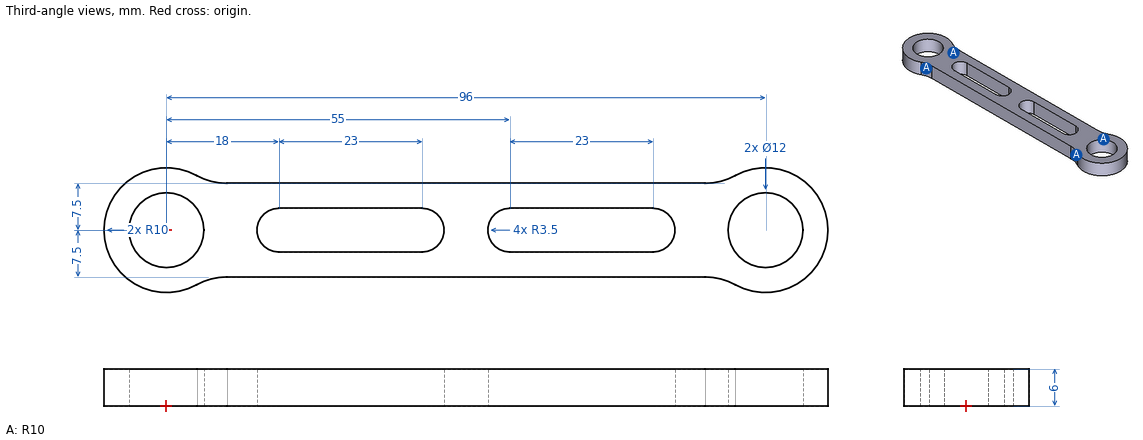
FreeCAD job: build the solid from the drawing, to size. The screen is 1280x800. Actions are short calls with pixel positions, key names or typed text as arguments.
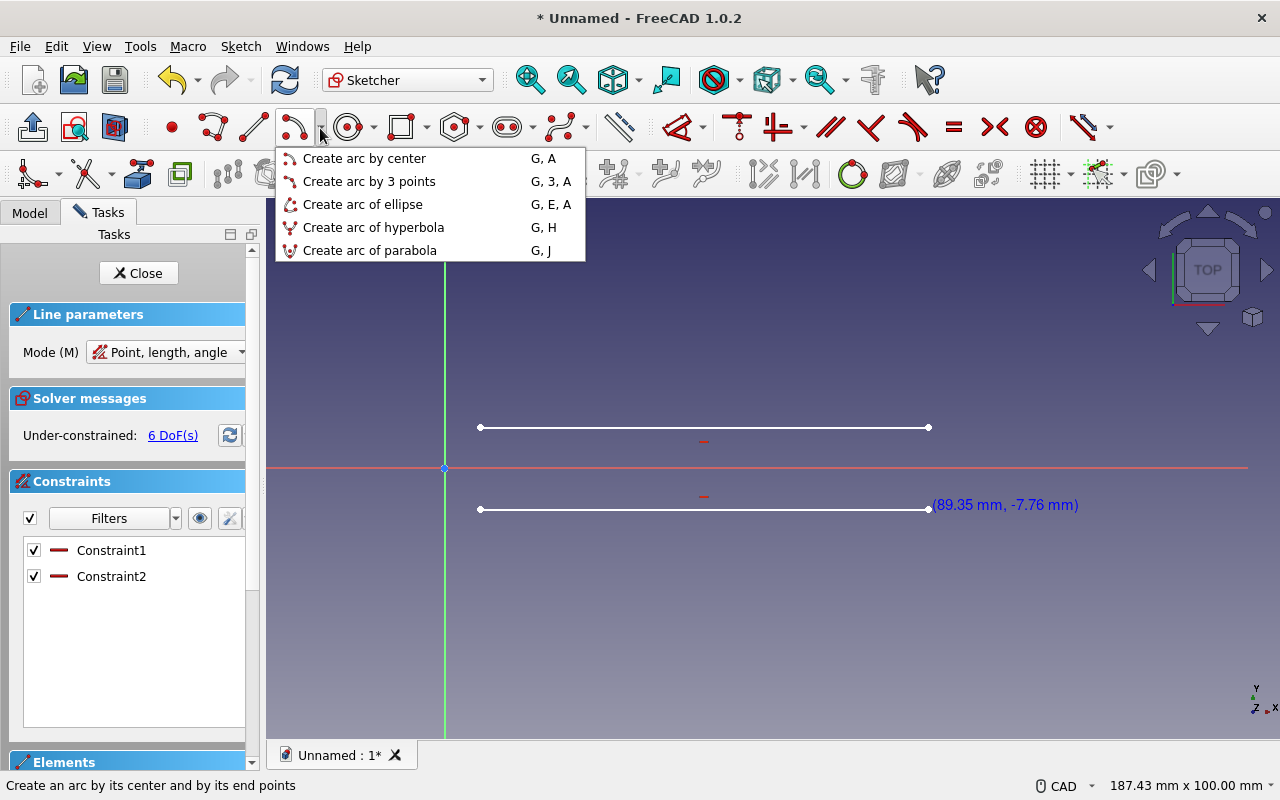
click(430, 182)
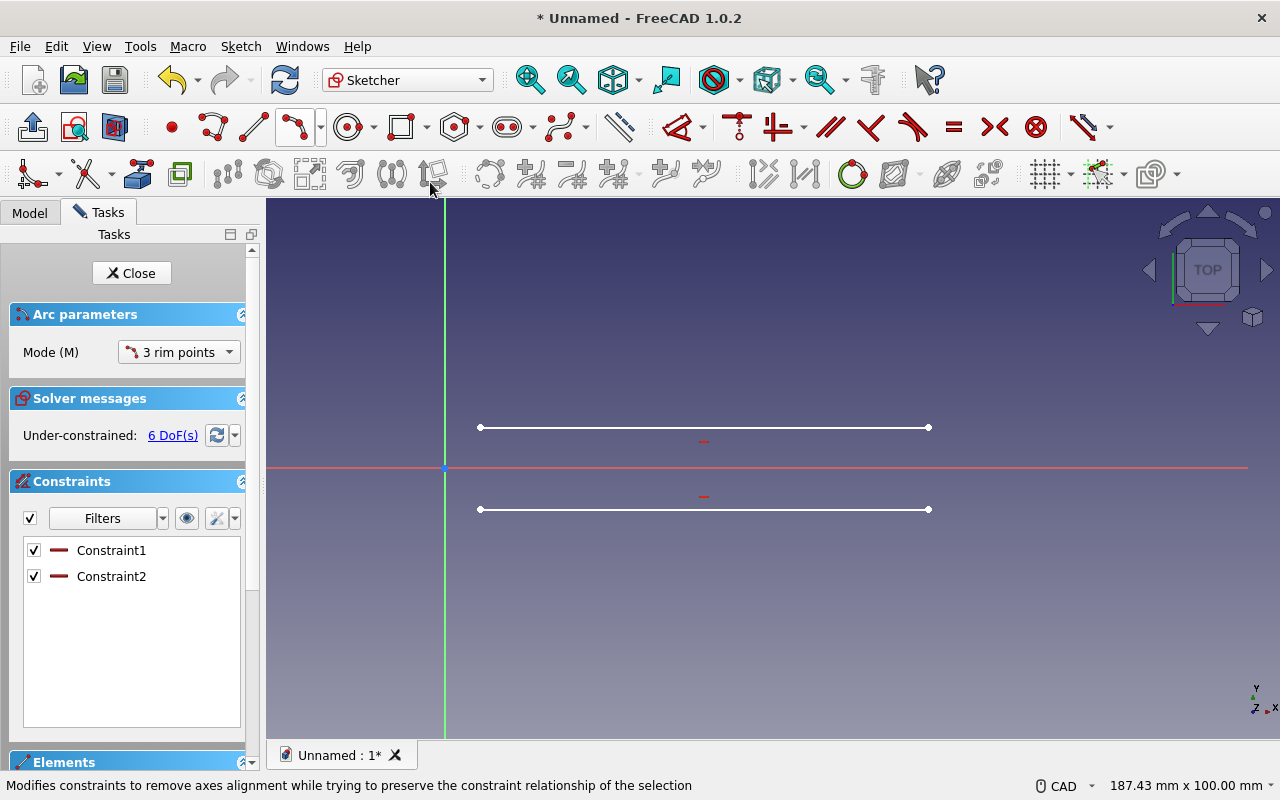
click(480, 428)
click(480, 510)
click(396, 444)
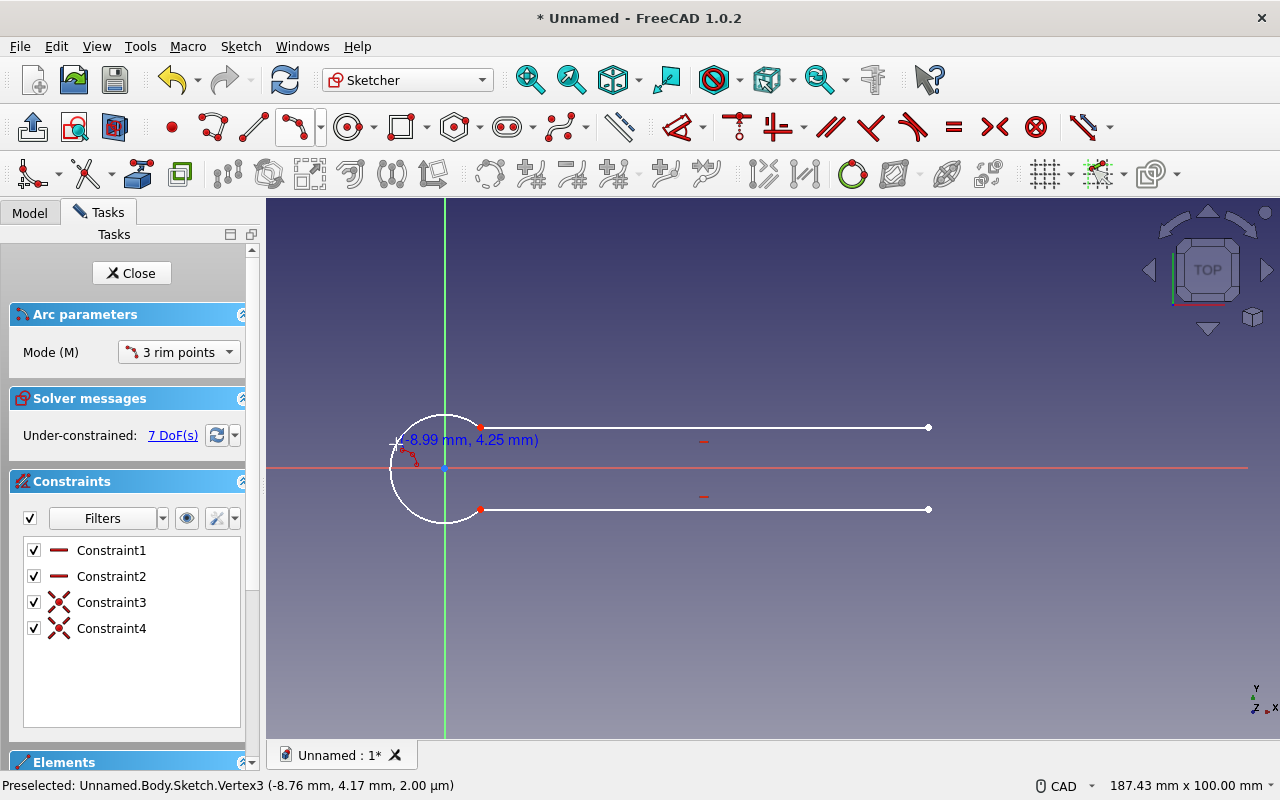
click(928, 510)
click(928, 428)
click(1012, 492)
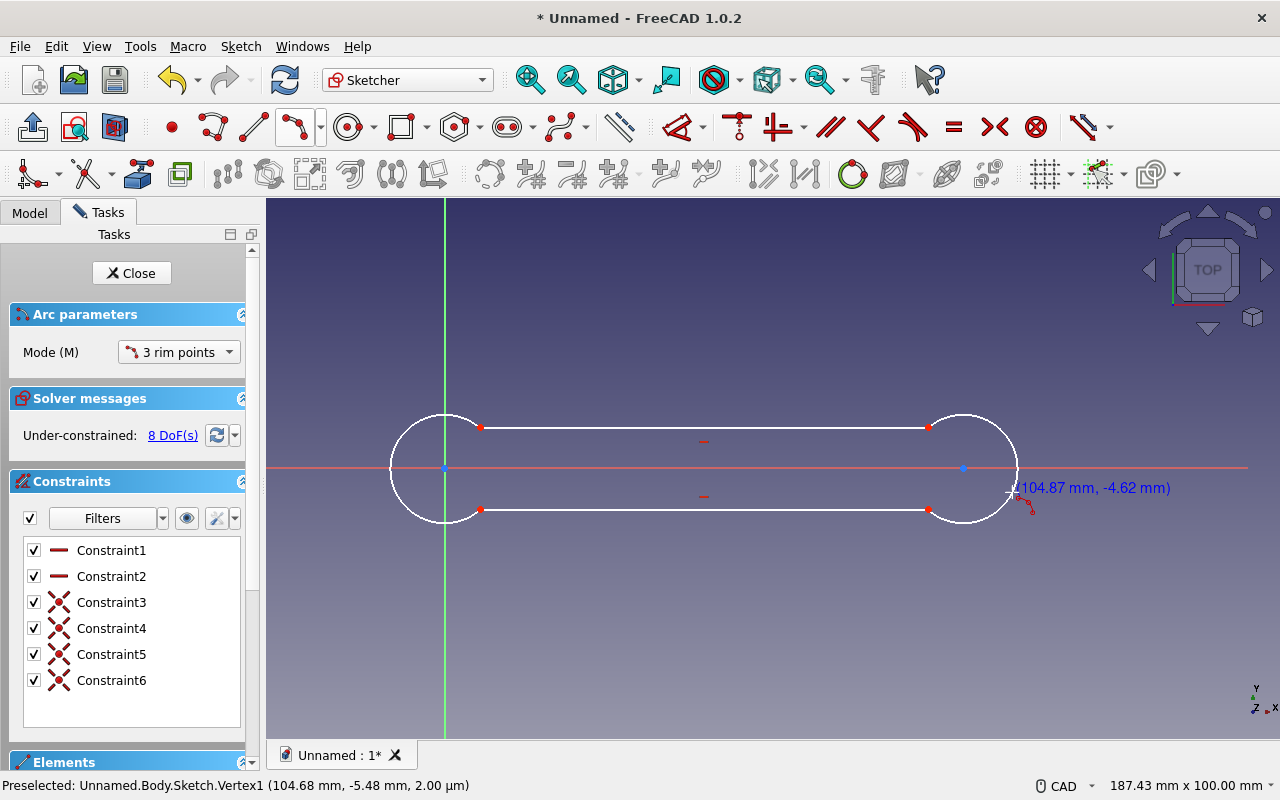
key(g)
key(s)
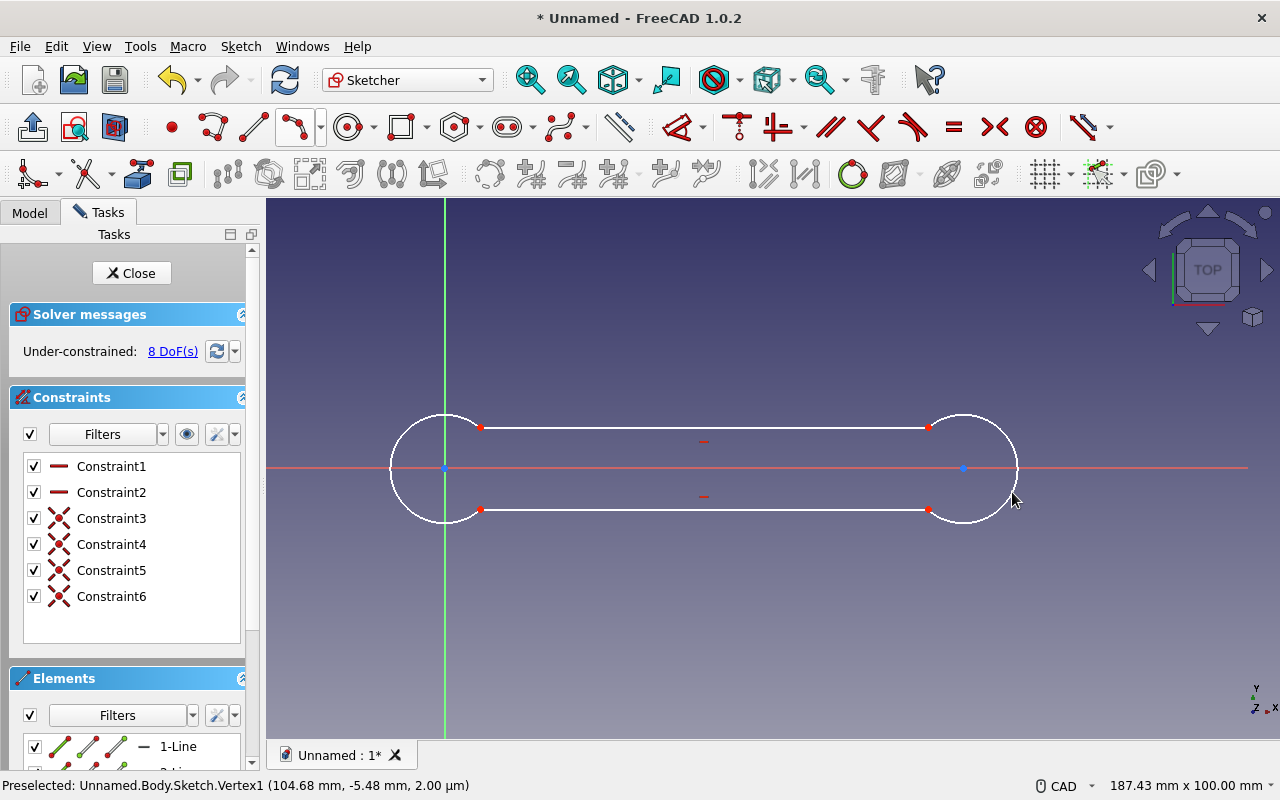
click(742, 468)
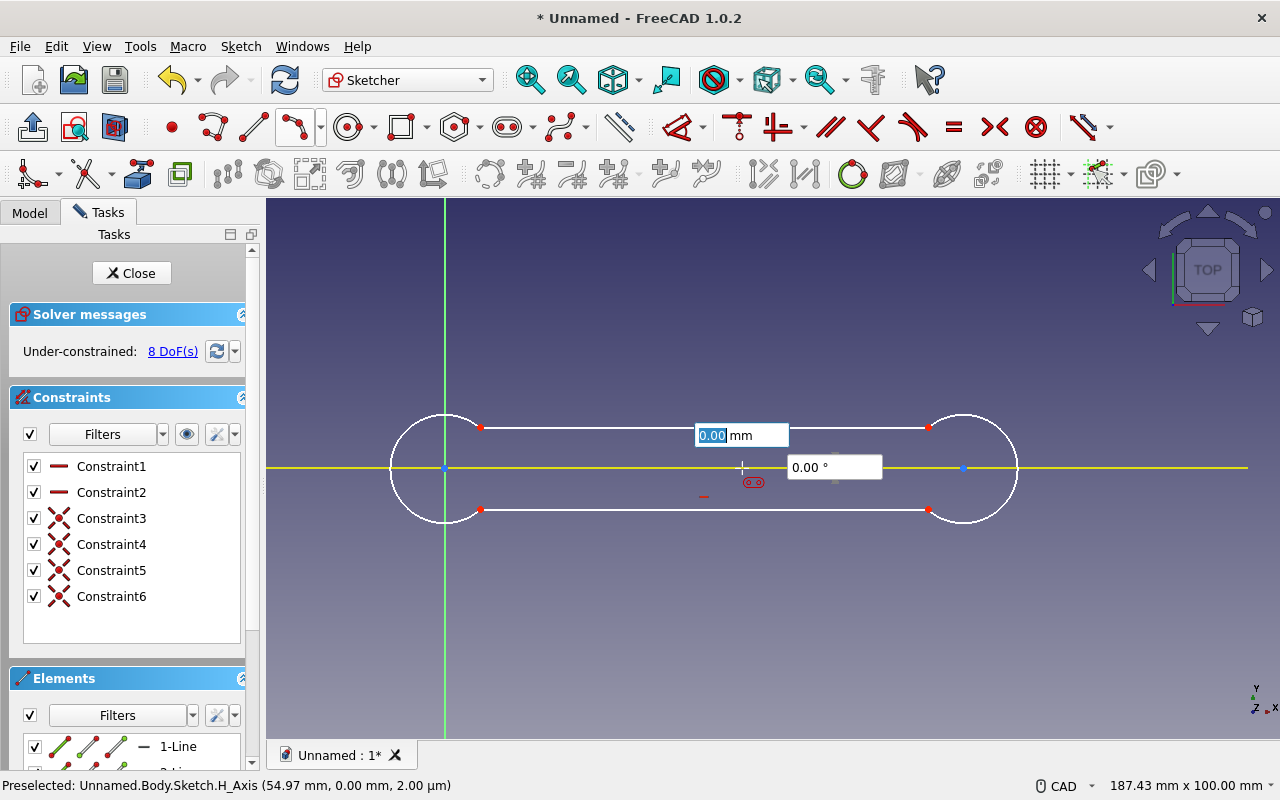
click(867, 459)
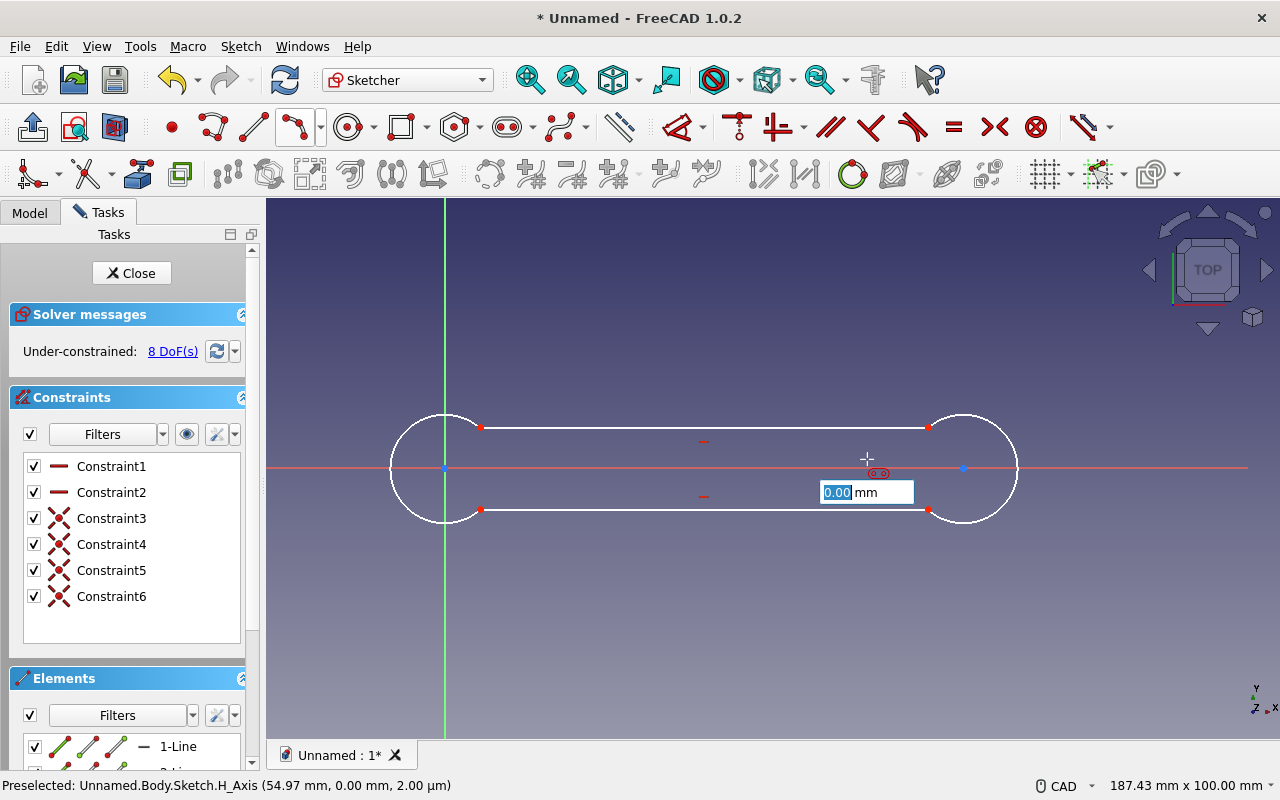
click(804, 487)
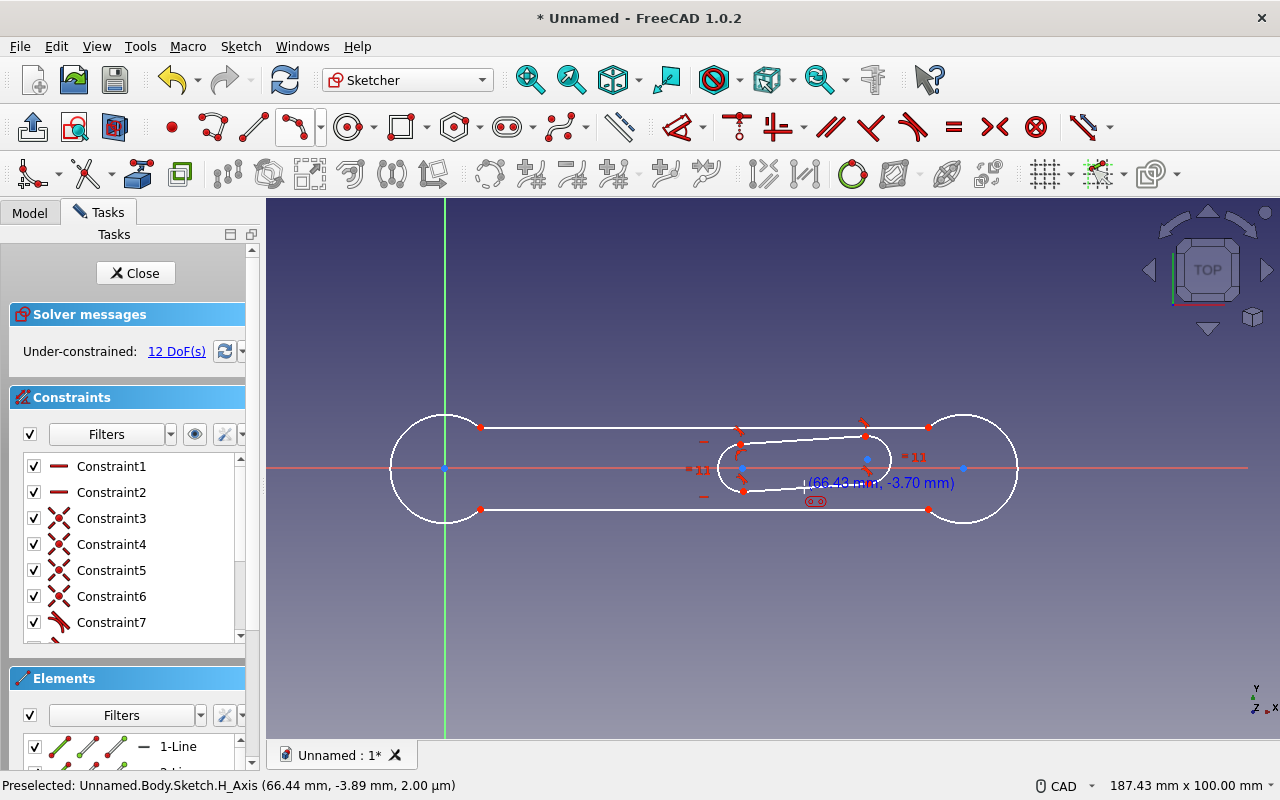
click(542, 468)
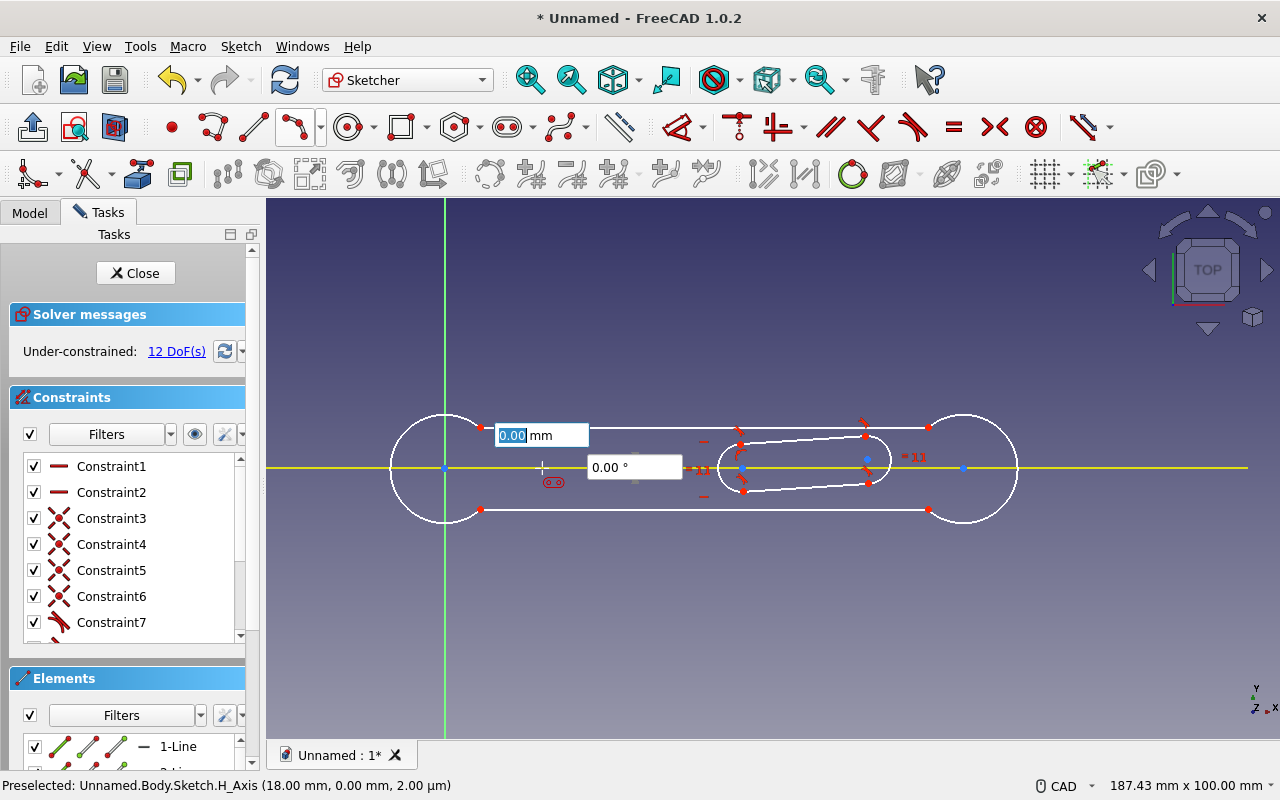
click(666, 459)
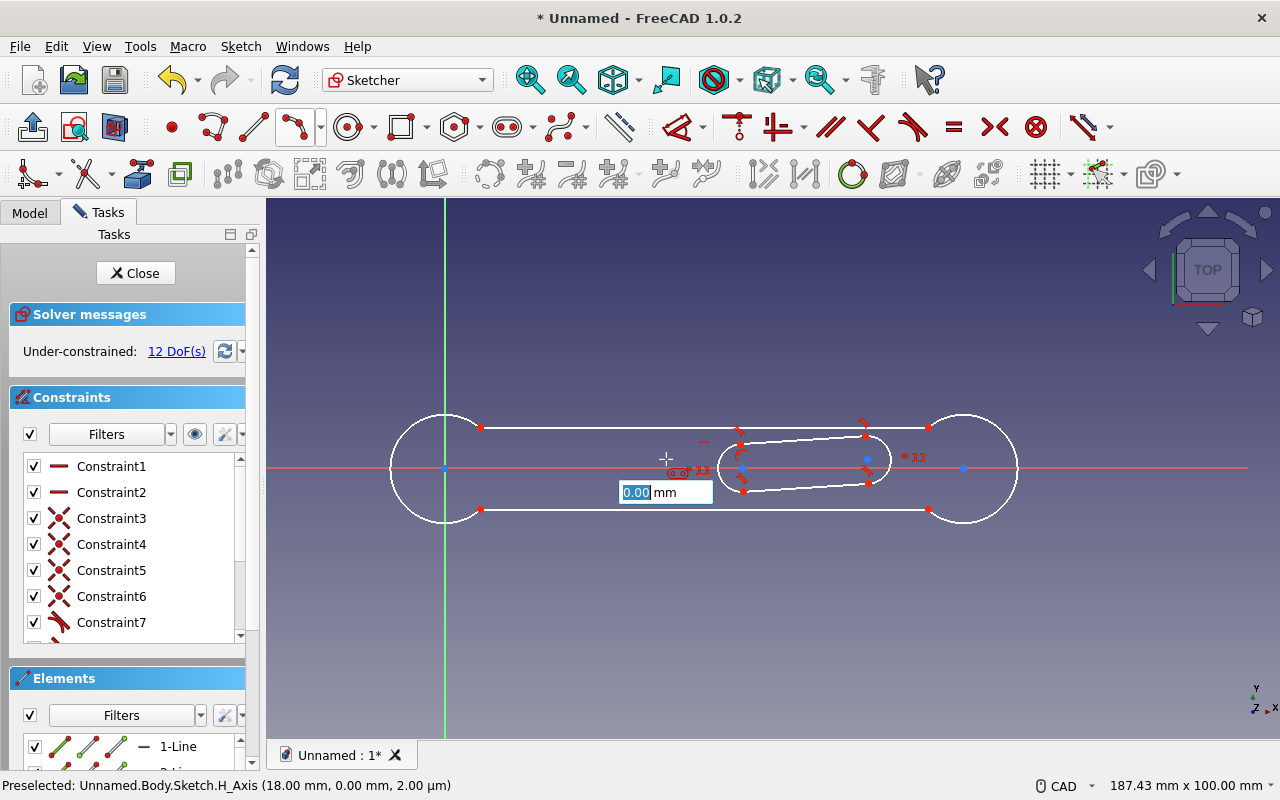
click(604, 449)